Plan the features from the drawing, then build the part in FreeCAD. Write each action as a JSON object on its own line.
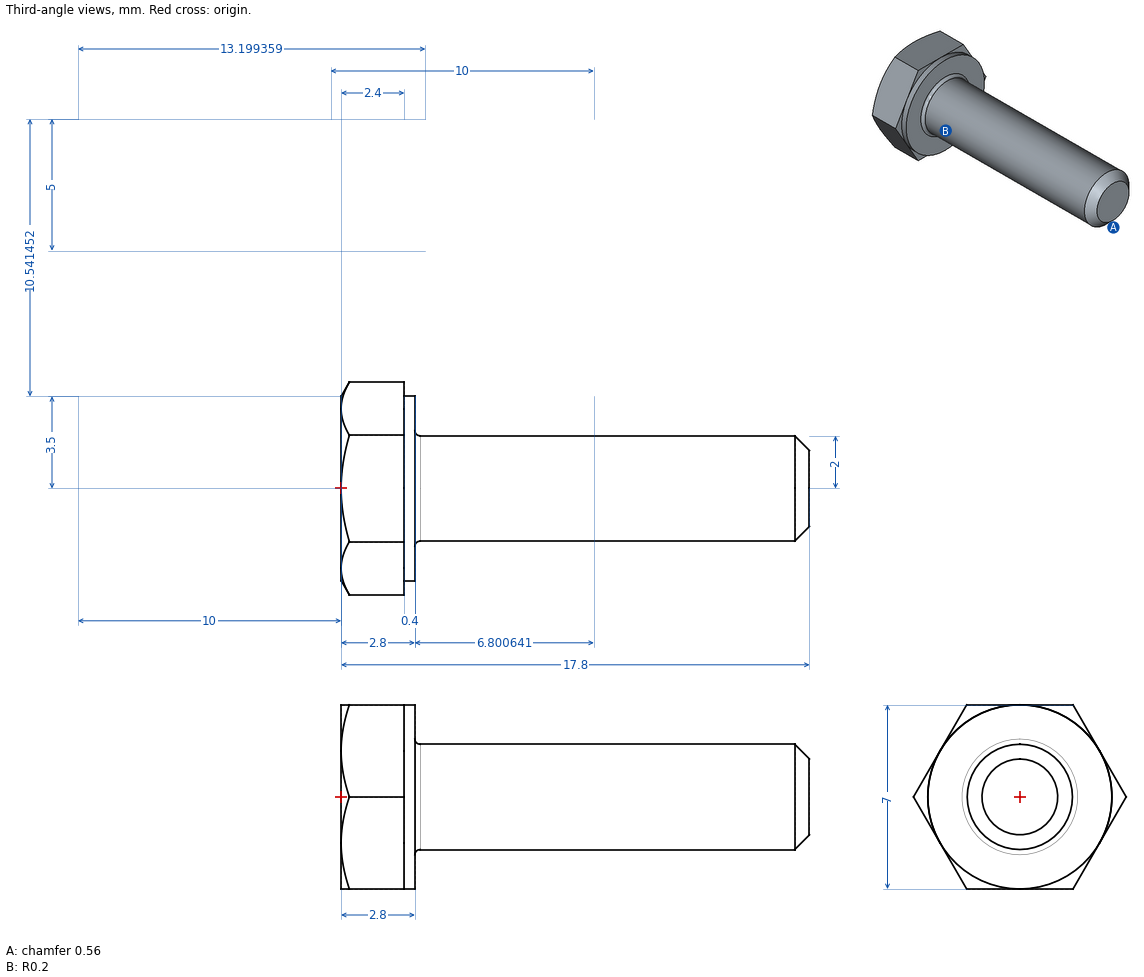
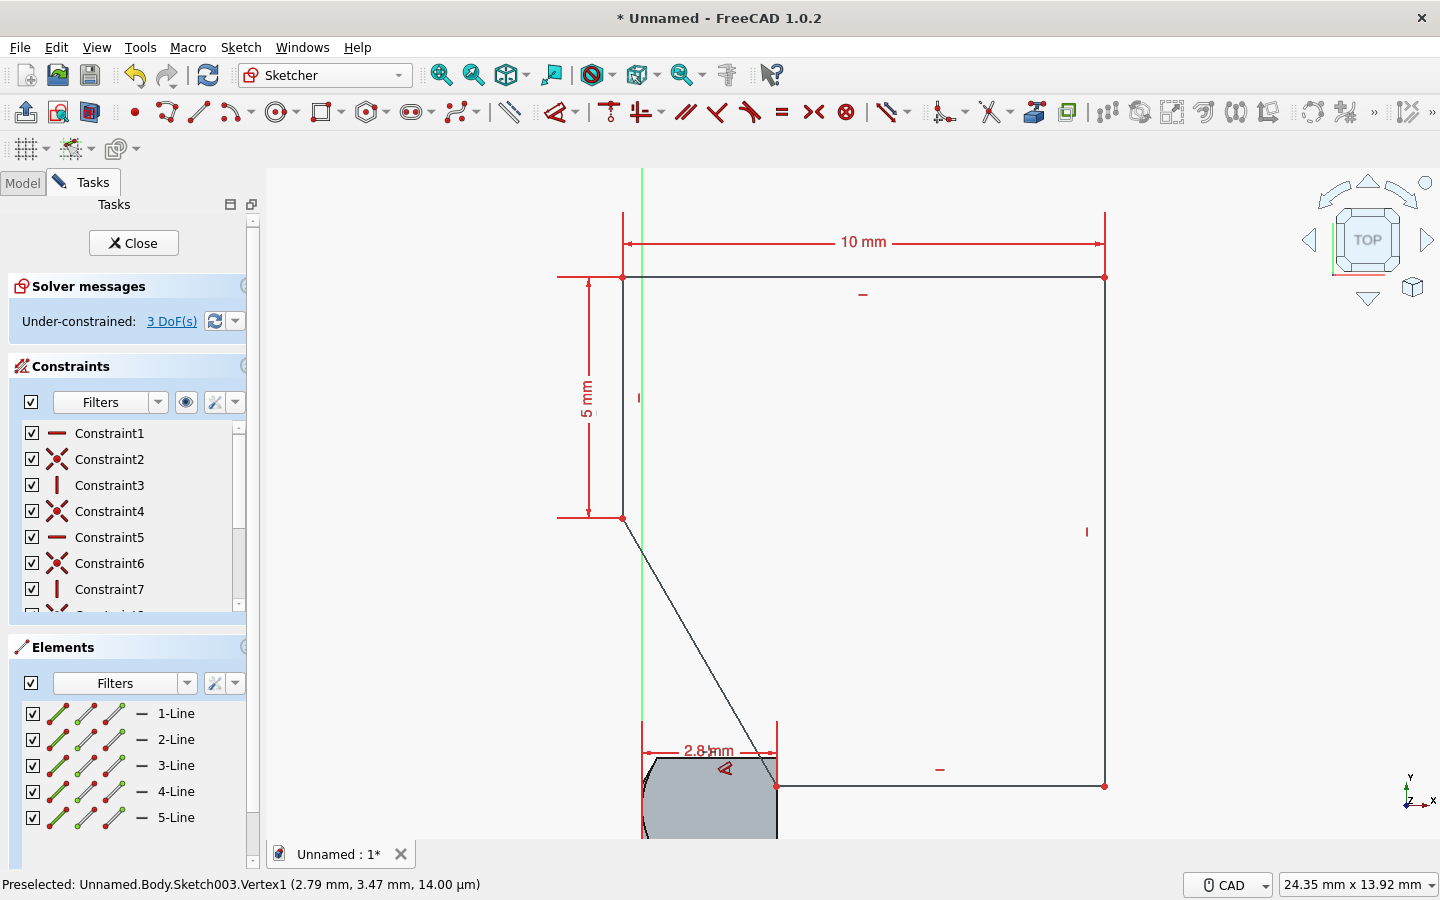
{"action": "left_click", "coordinate": [777, 786]}
{"action": "left_click", "coordinate": [608, 799]}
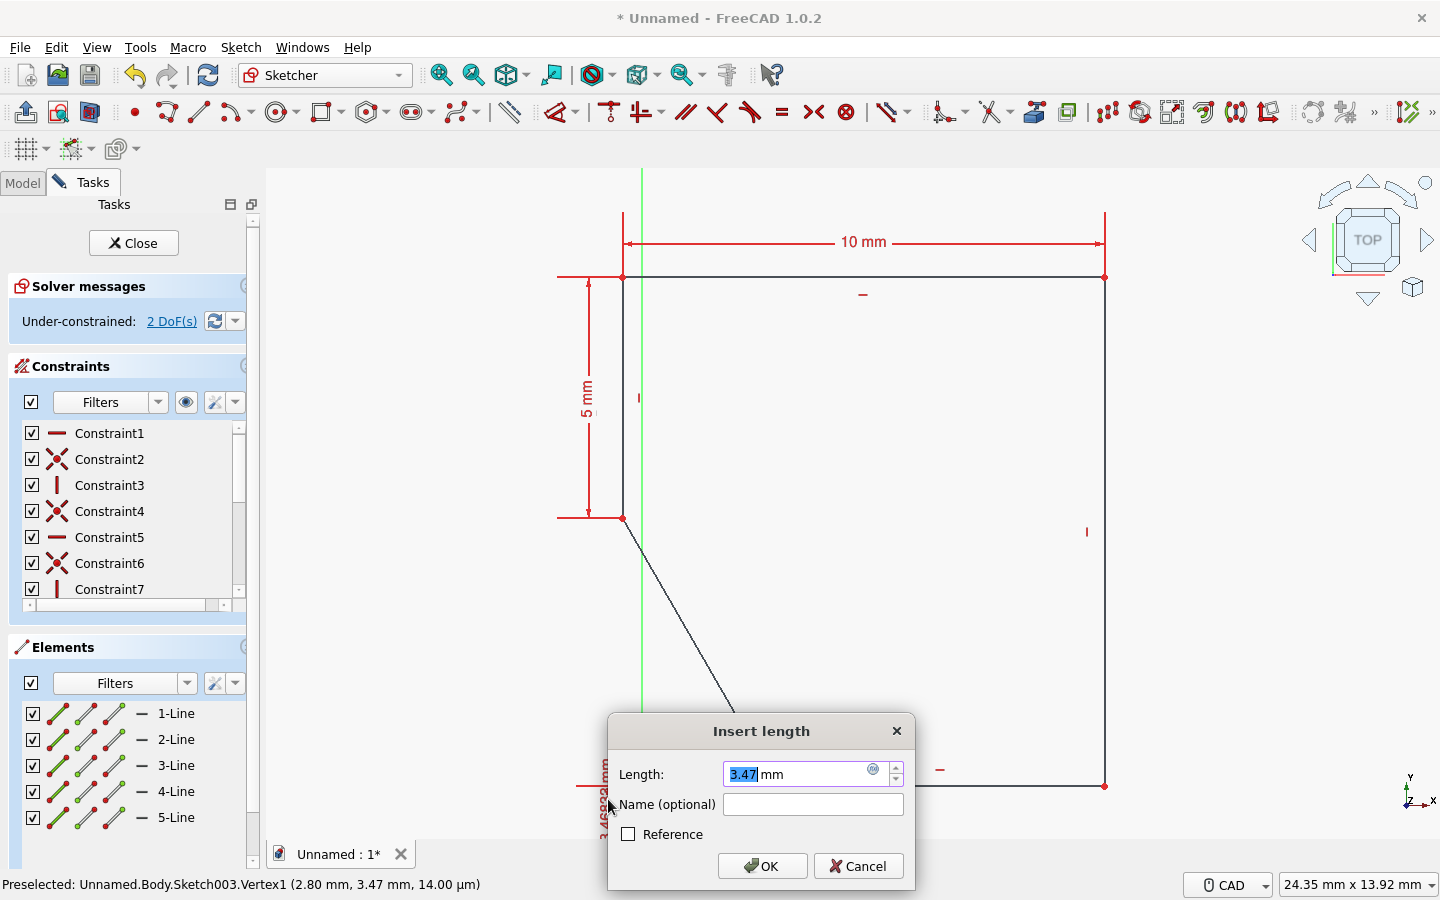
{"action": "type", "text": "3.5"}
{"action": "key", "text": "Return"}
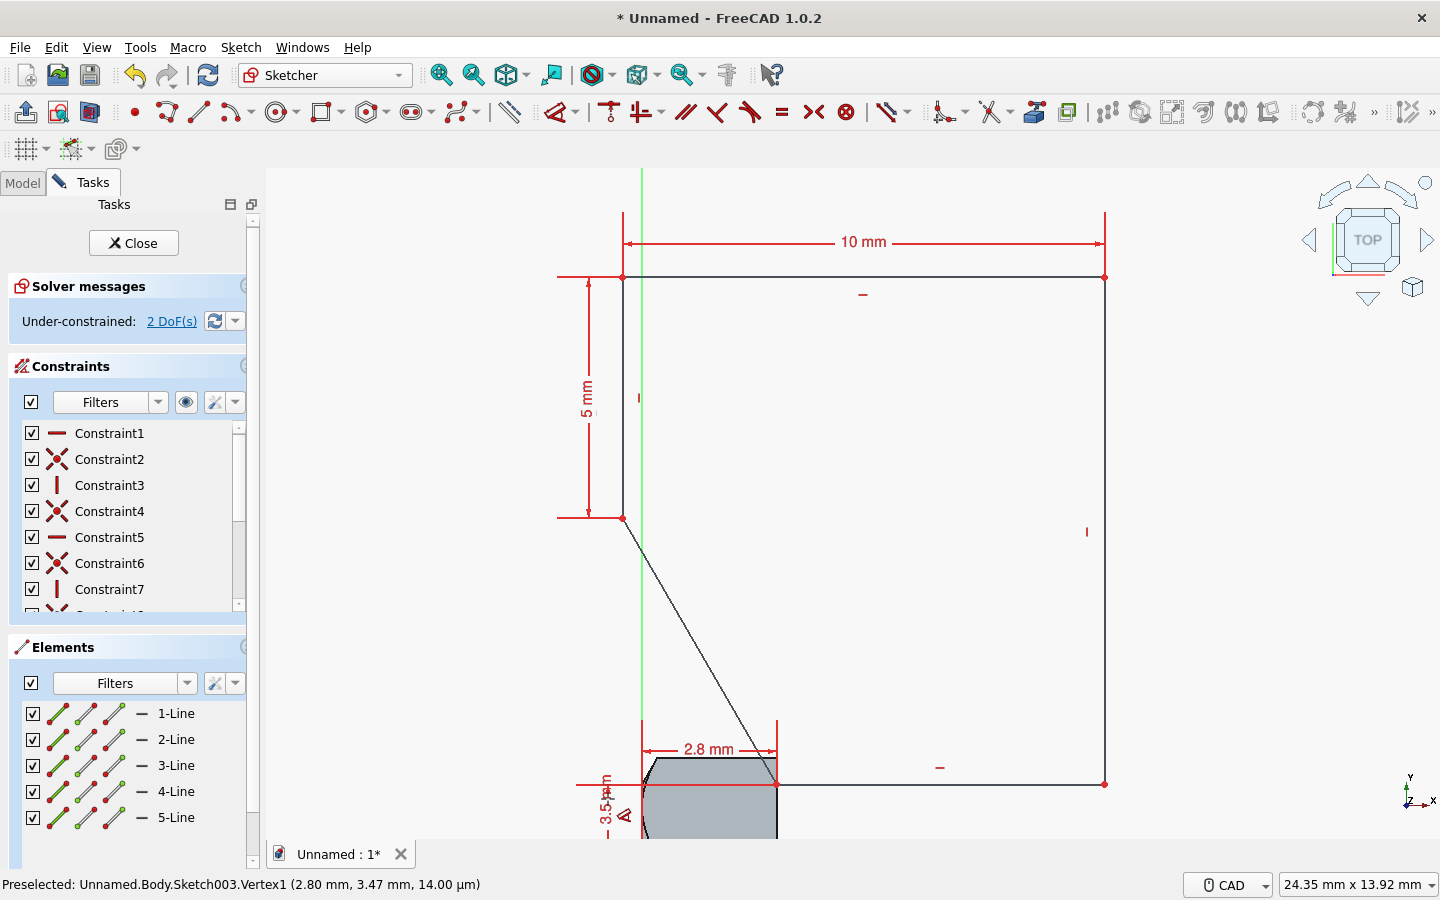
{"action": "left_click", "coordinate": [875, 785]}
{"action": "left_click", "coordinate": [941, 751]}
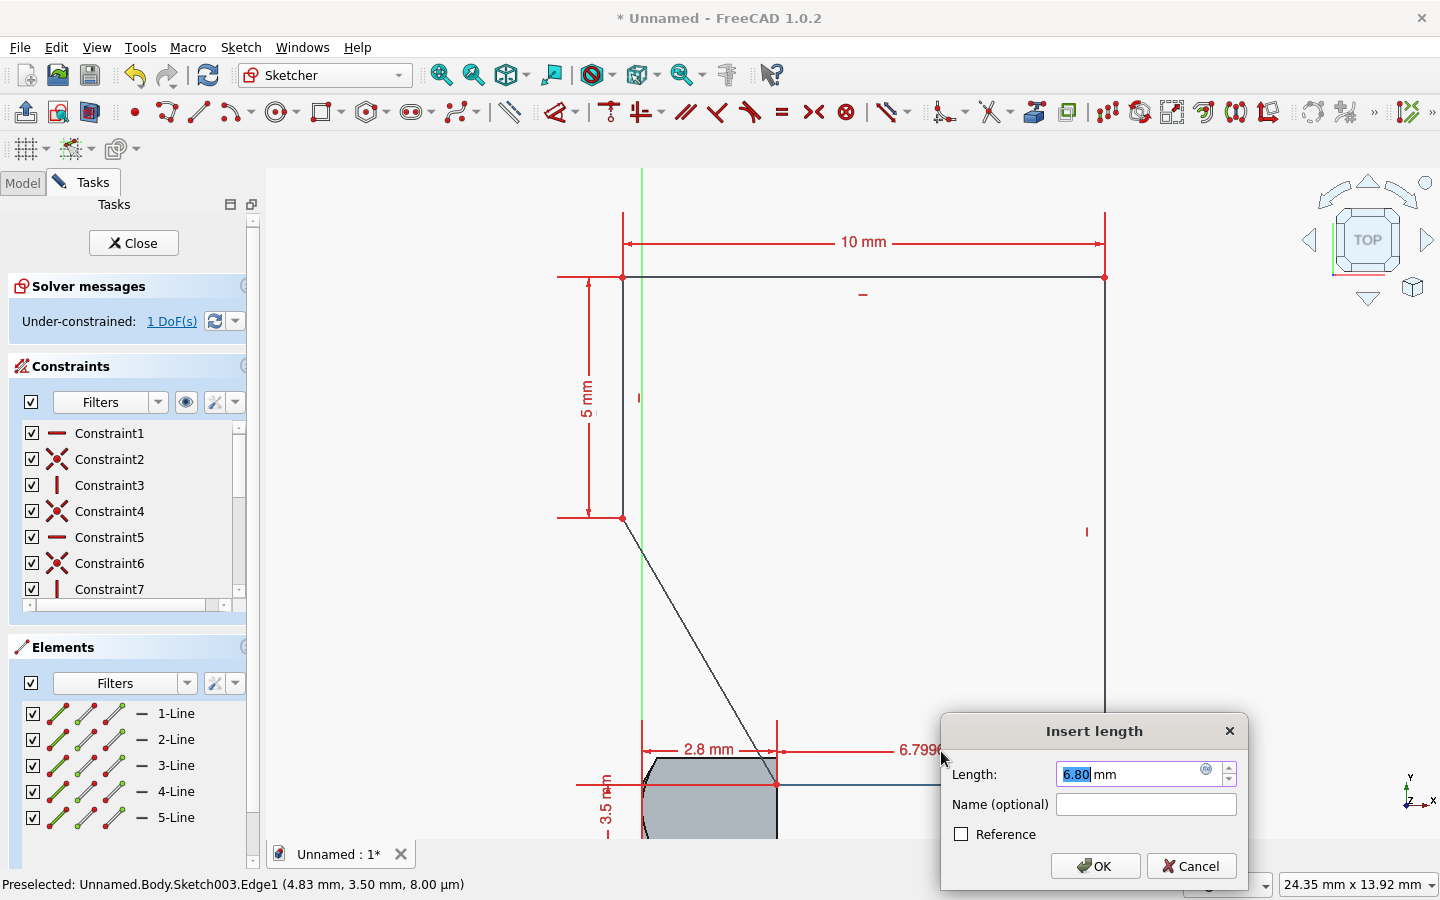
{"action": "type", "text": "6.800641"}
{"action": "key", "text": "Return"}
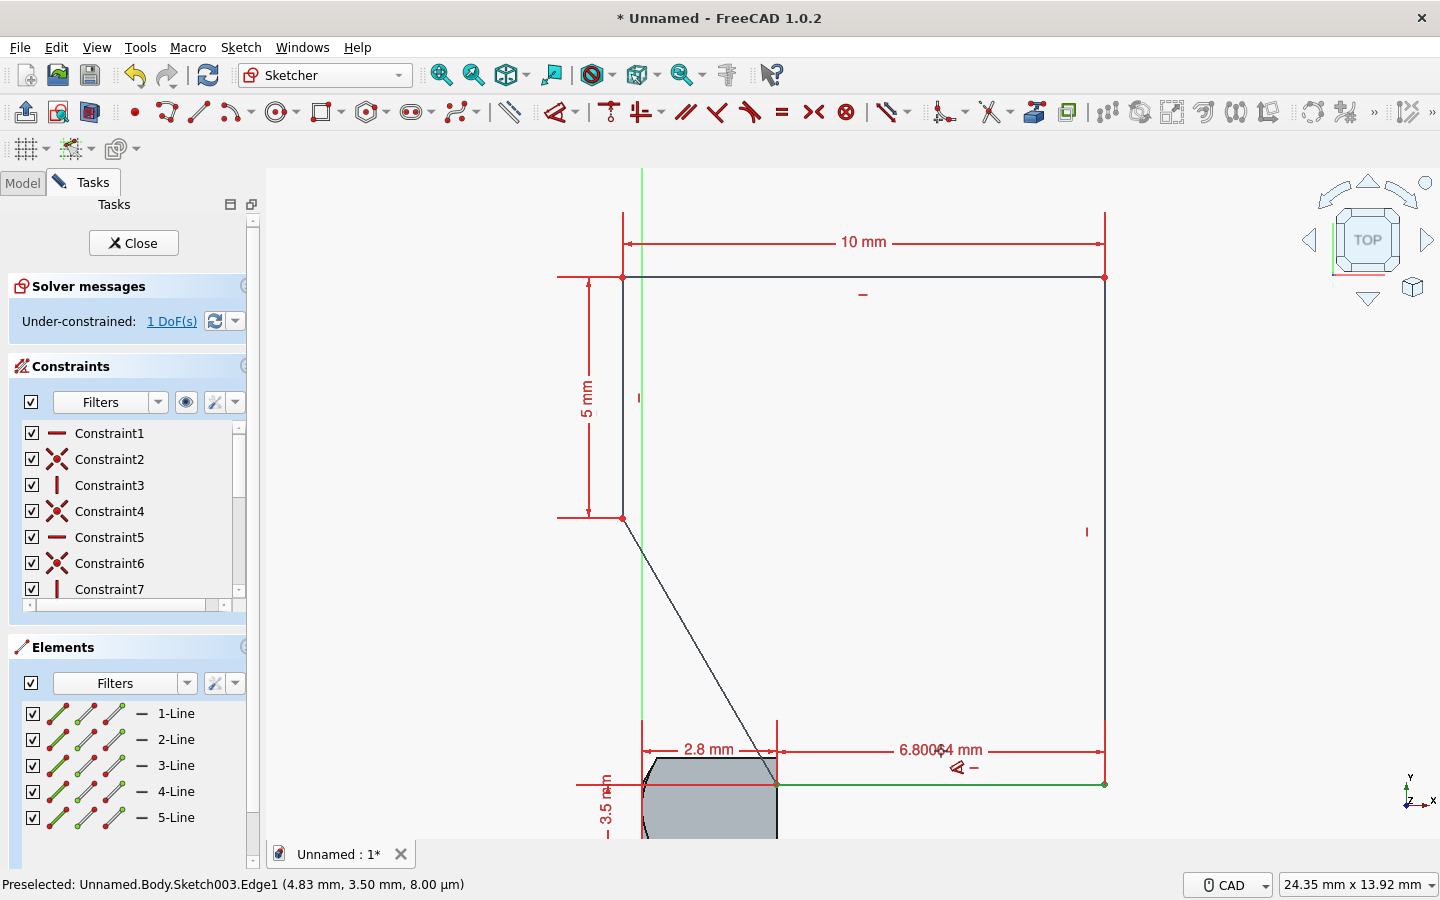
{"action": "left_click", "coordinate": [1105, 632]}
{"action": "left_click", "coordinate": [1139, 531]}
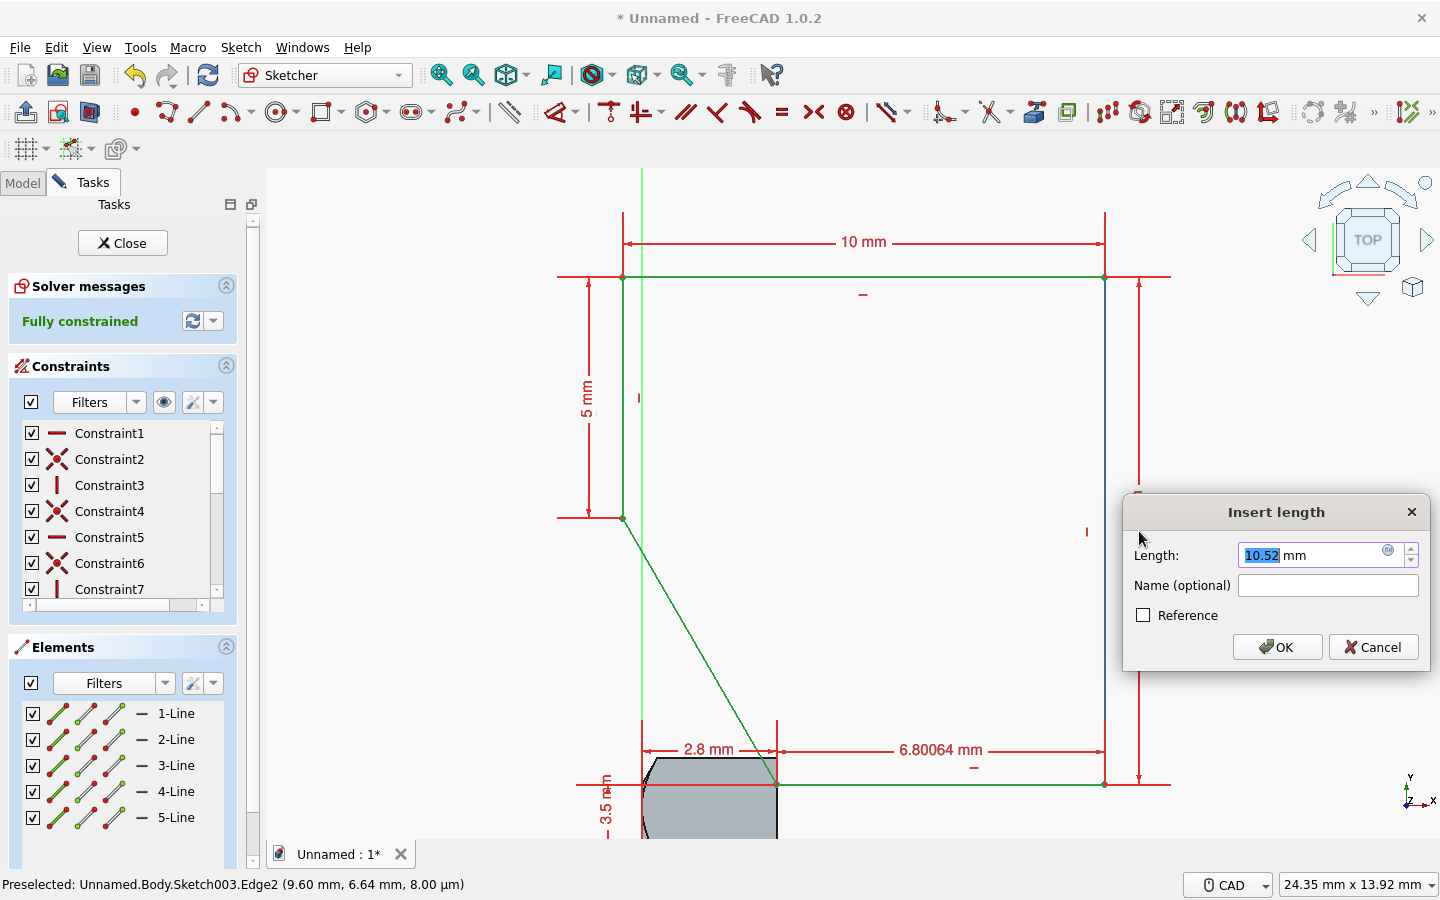
{"action": "type", "text": "10.541452"}
{"action": "key", "text": "Return"}
{"action": "key", "text": "Escape"}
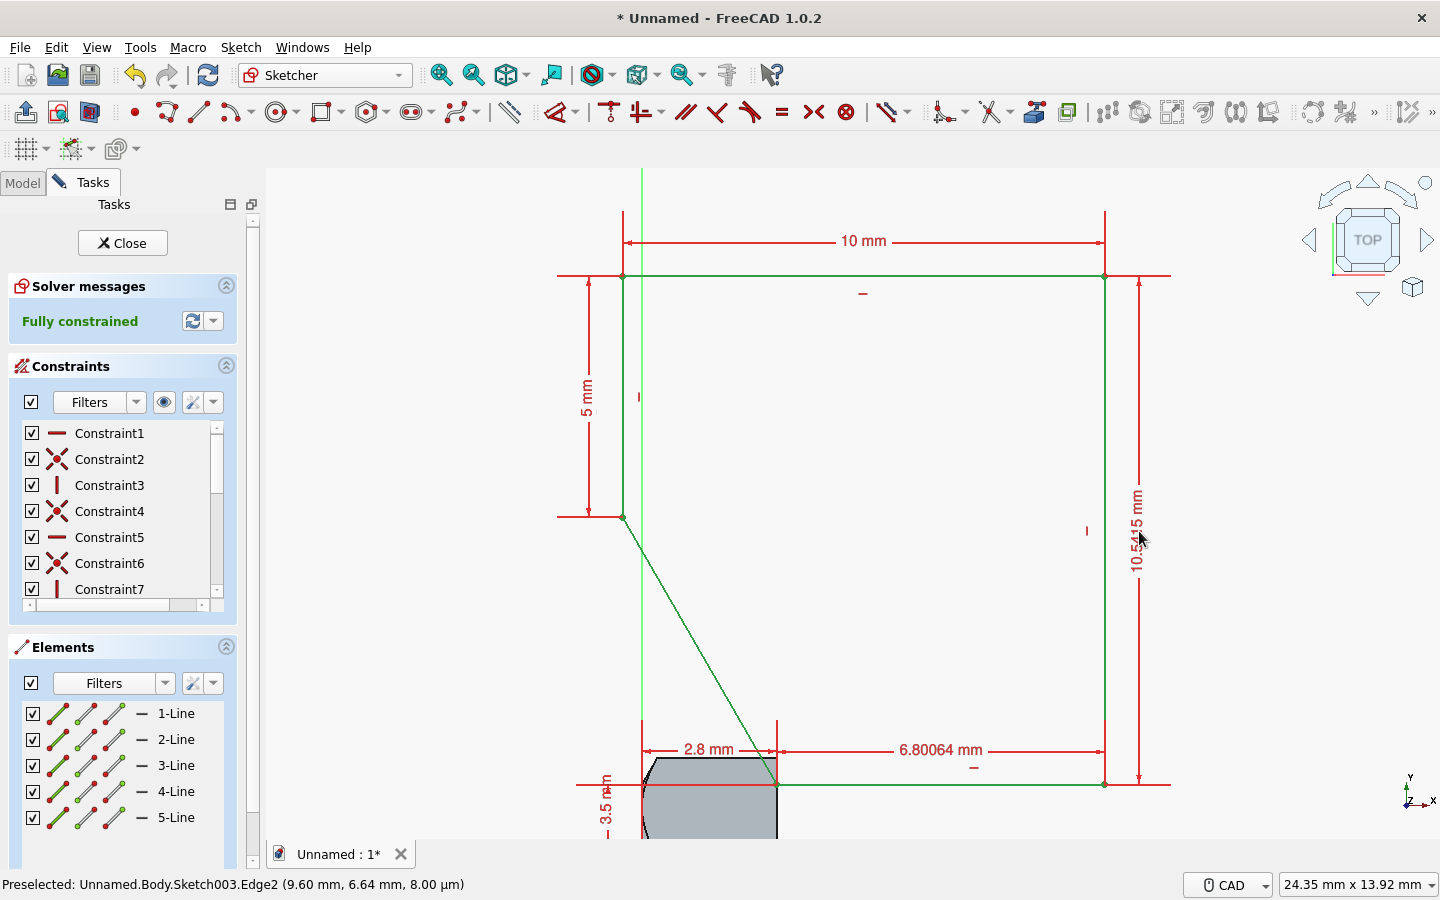
{"action": "left_click", "coordinate": [123, 243]}